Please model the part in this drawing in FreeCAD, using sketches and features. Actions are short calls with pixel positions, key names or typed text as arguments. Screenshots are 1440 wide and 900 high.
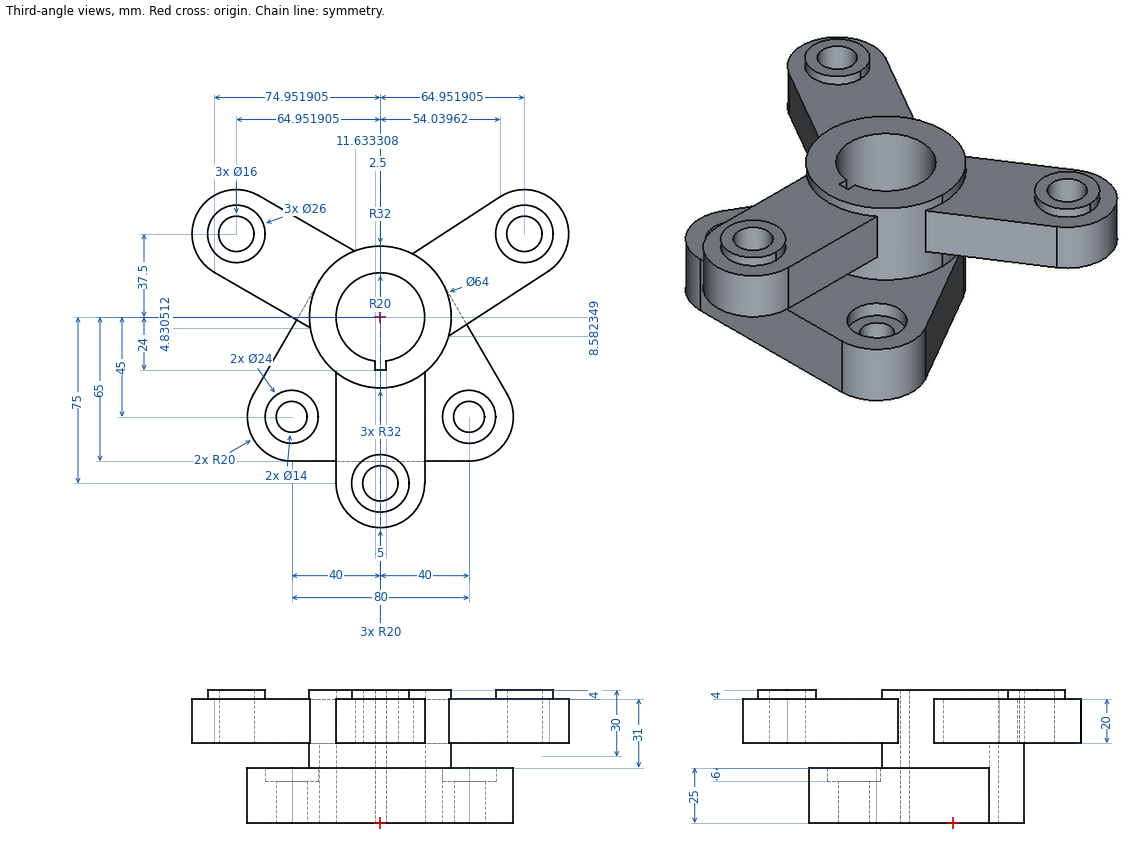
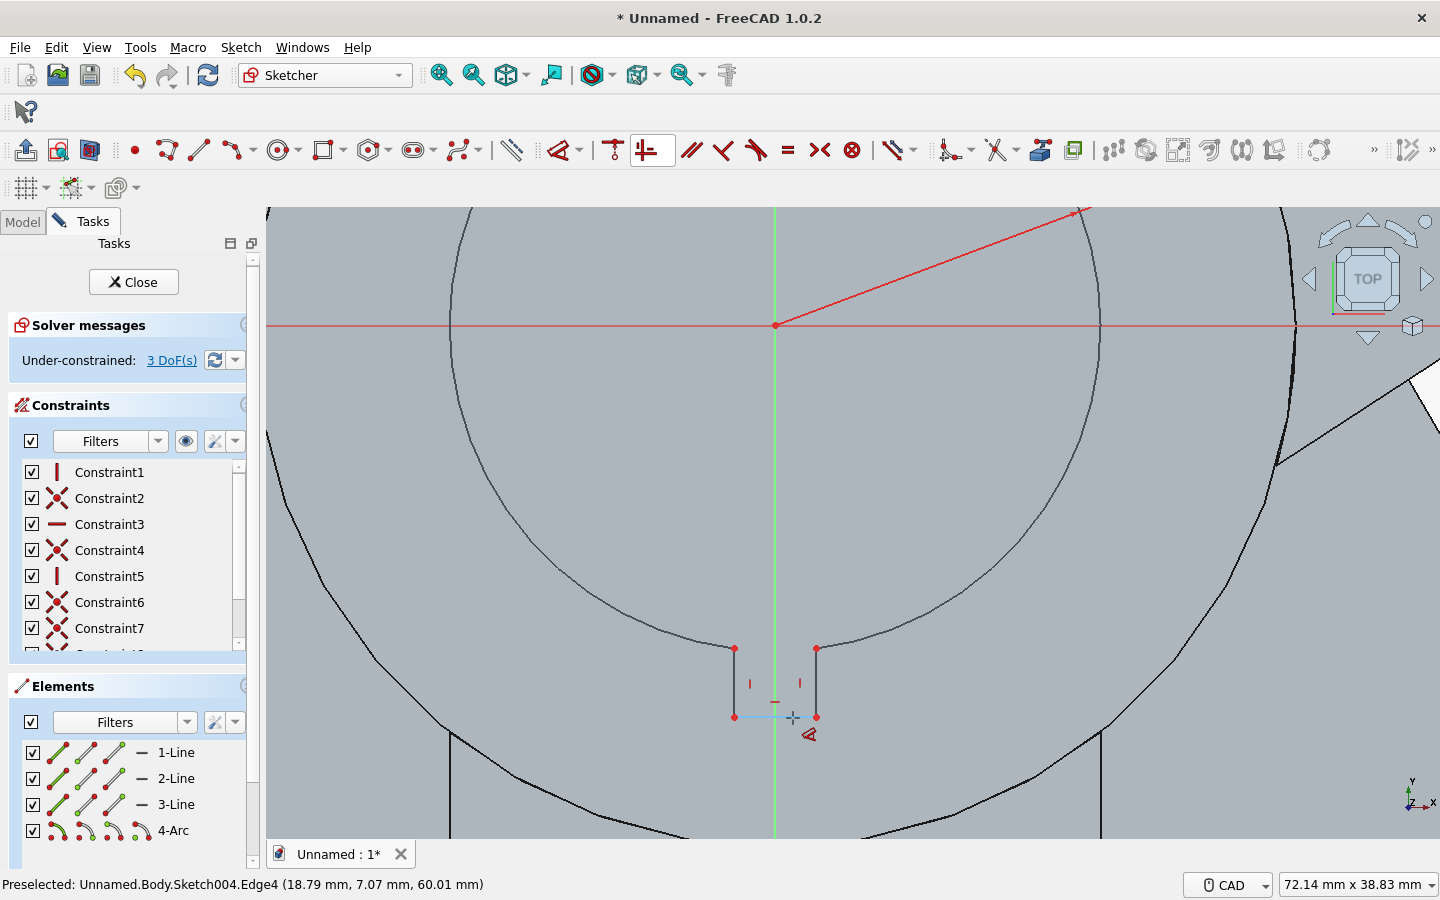
click(792, 717)
click(756, 751)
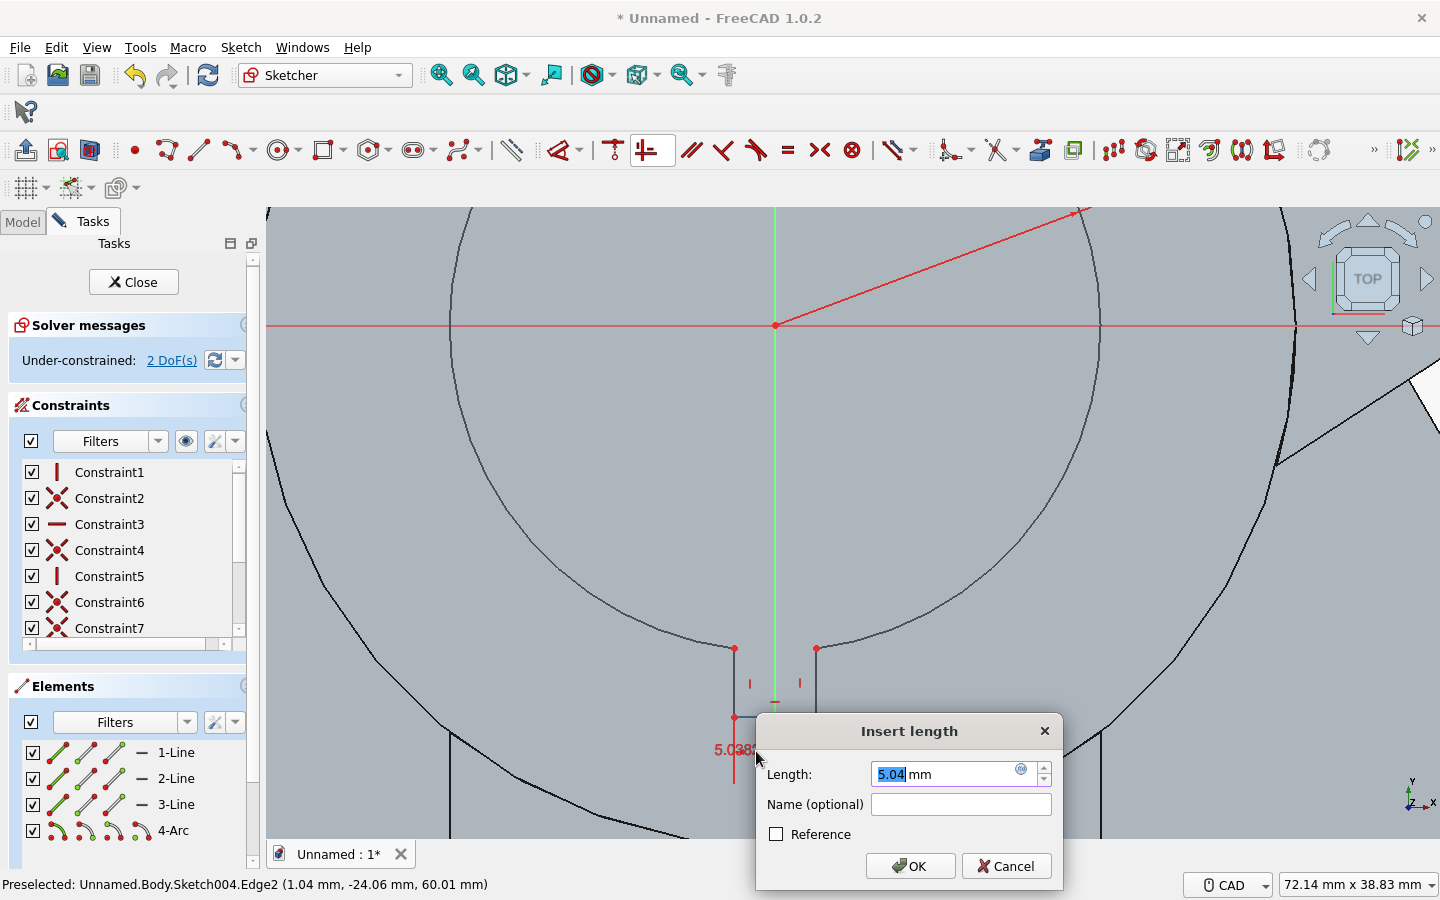
text(5)
key(Return)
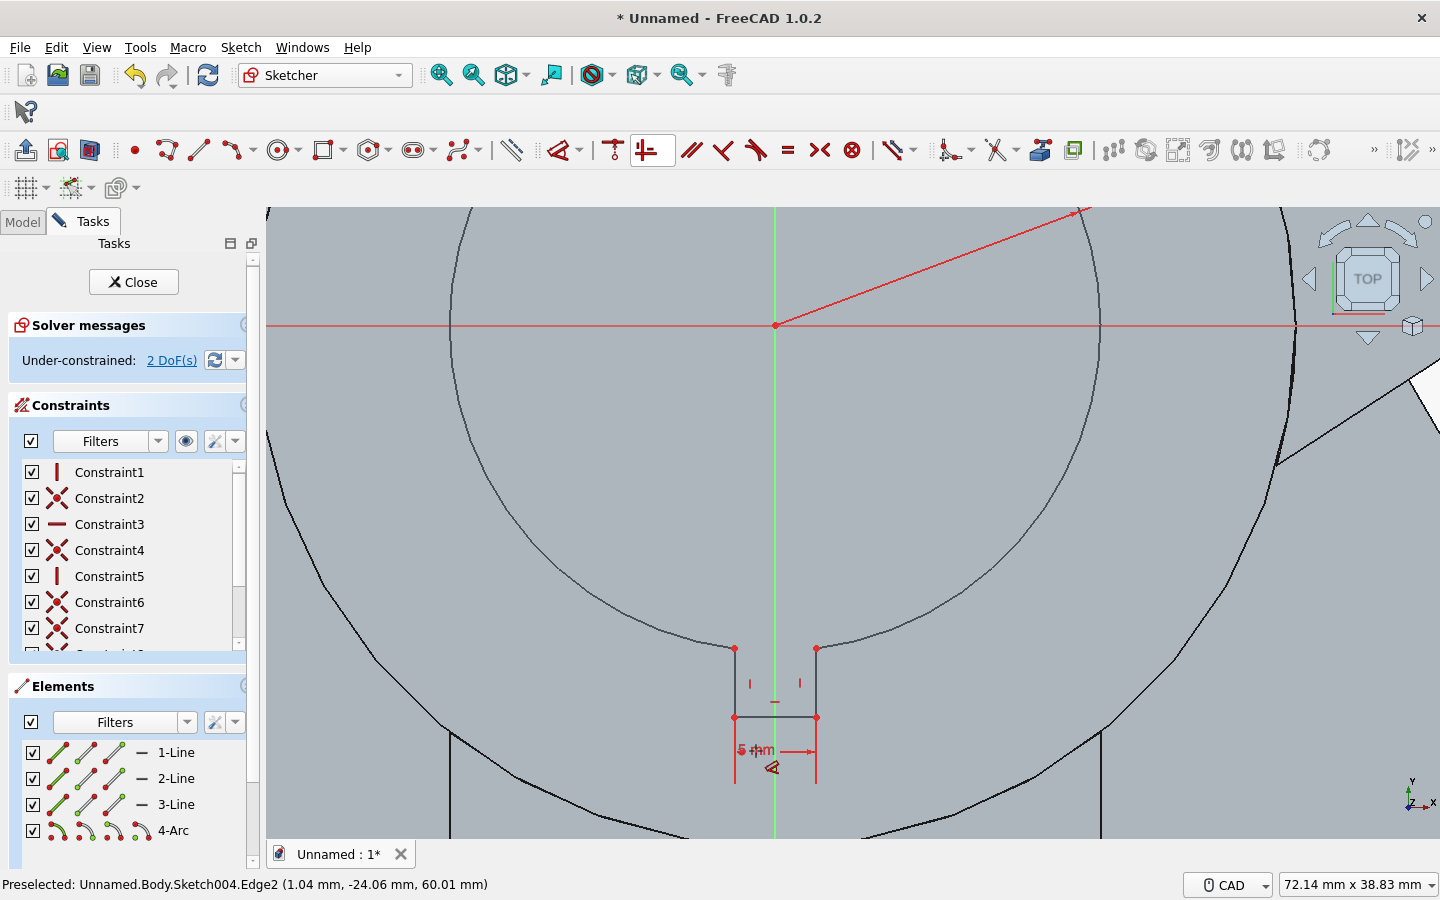
click(735, 717)
click(701, 522)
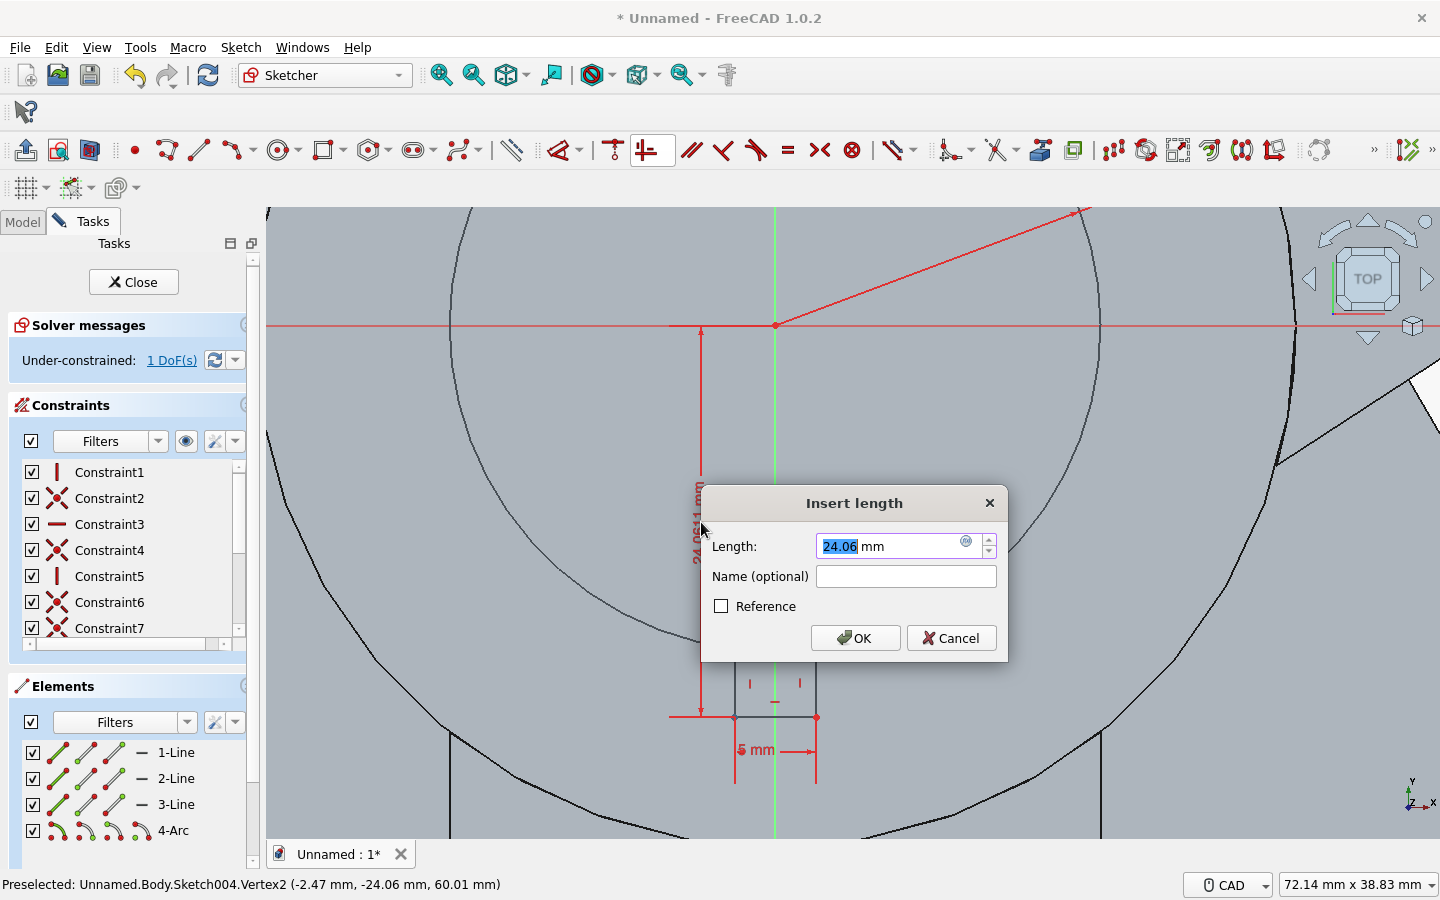
text(24)
key(Return)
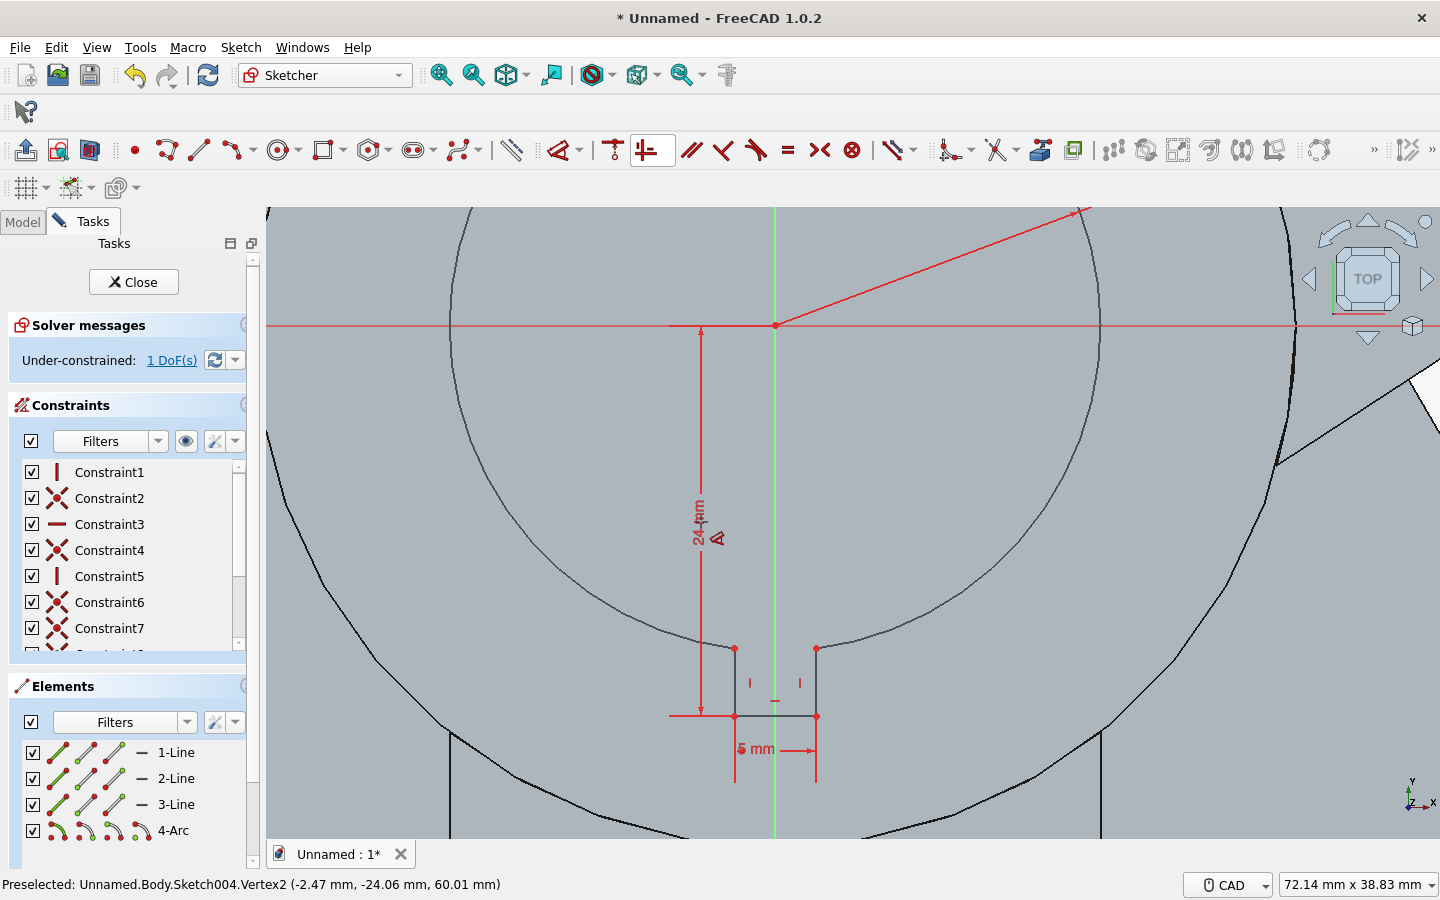
click(735, 649)
click(755, 683)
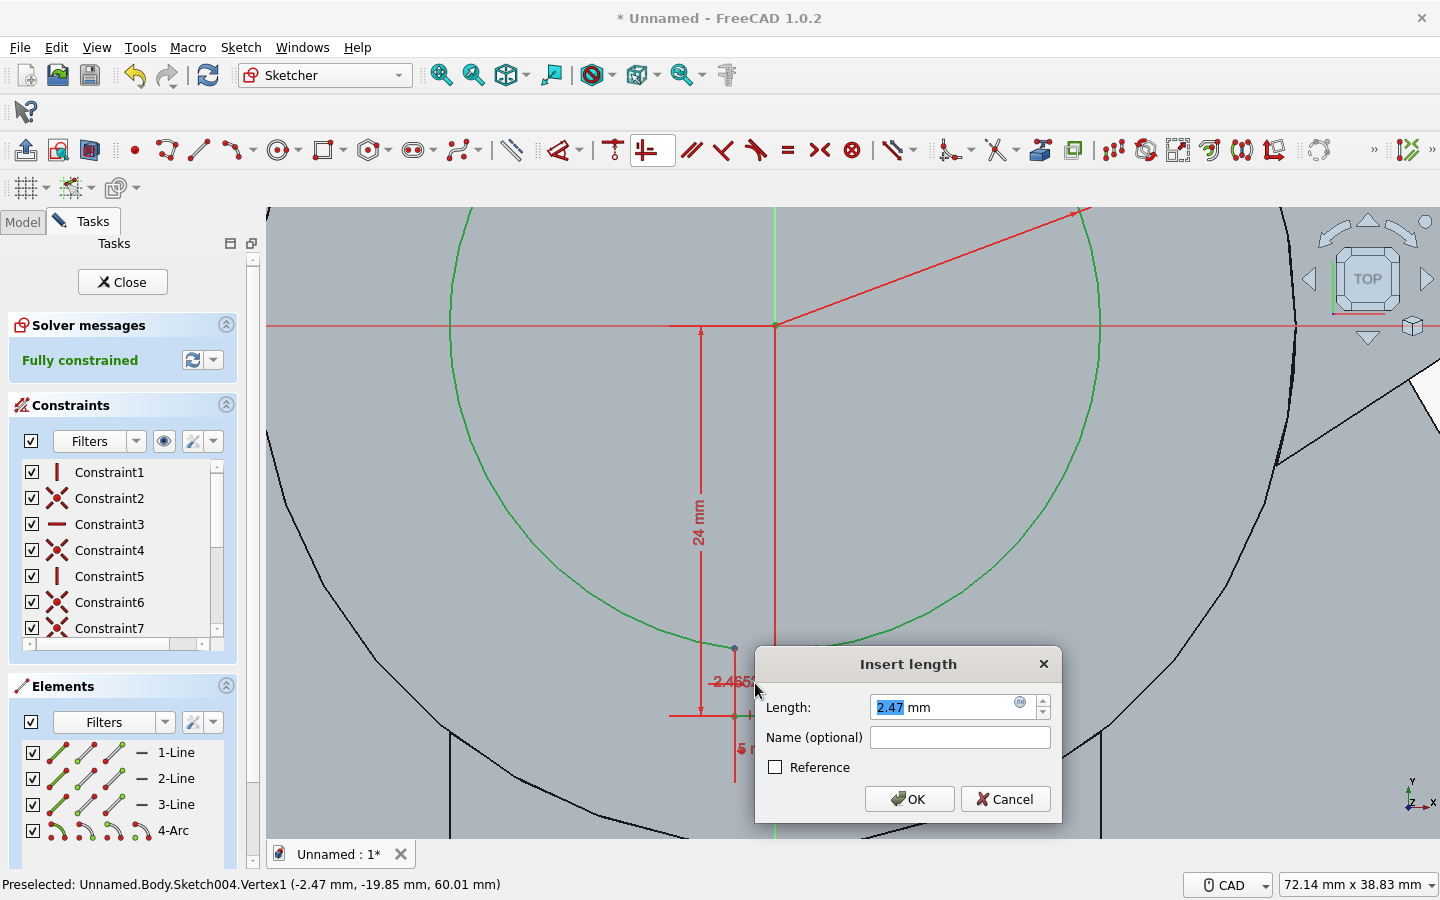
text(2.5)
key(Return)
key(Escape)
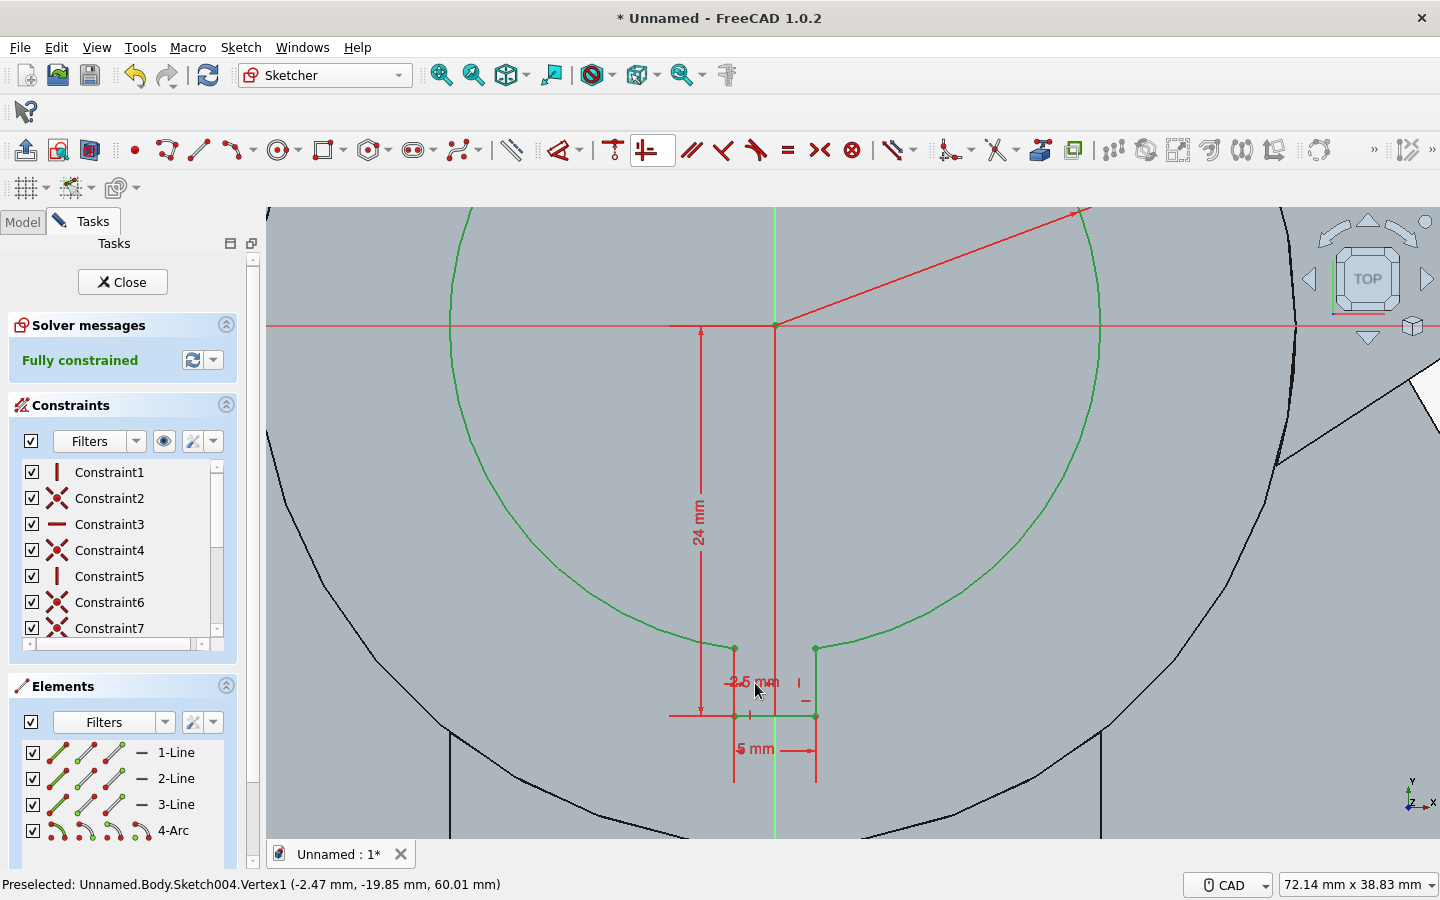
click(123, 282)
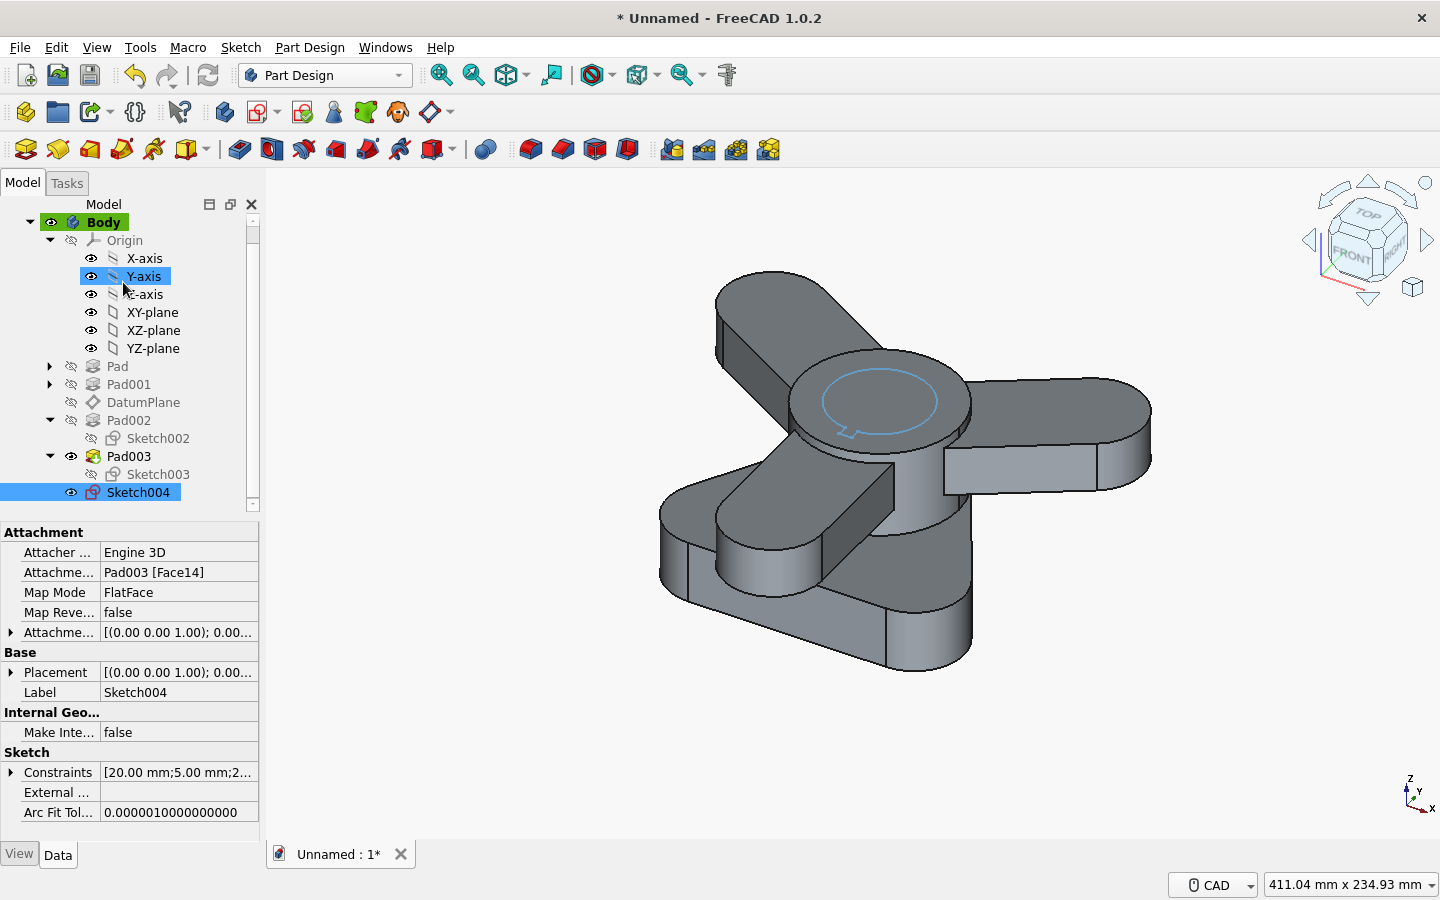
click(240, 150)